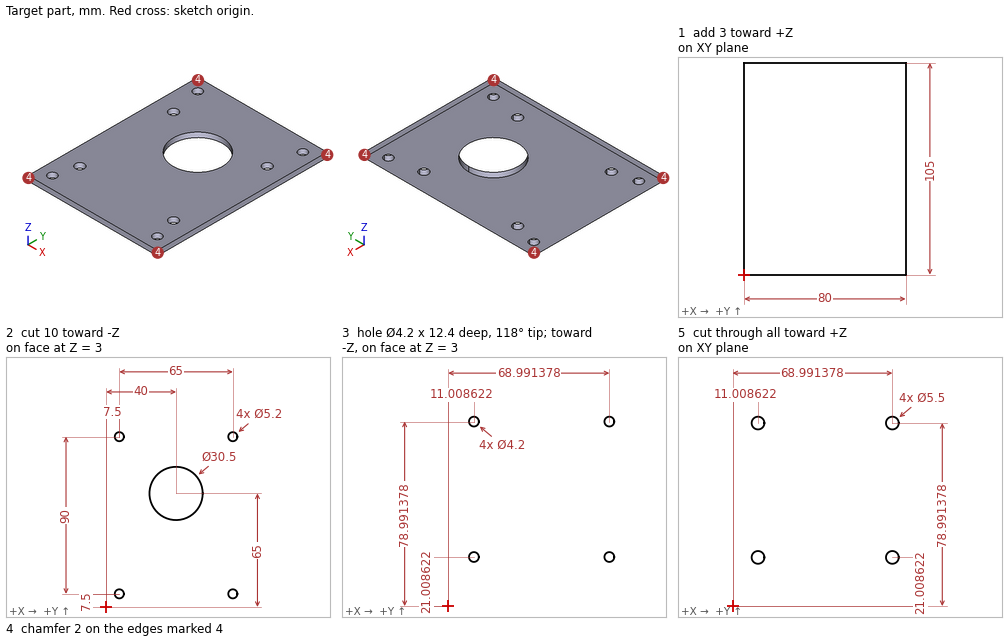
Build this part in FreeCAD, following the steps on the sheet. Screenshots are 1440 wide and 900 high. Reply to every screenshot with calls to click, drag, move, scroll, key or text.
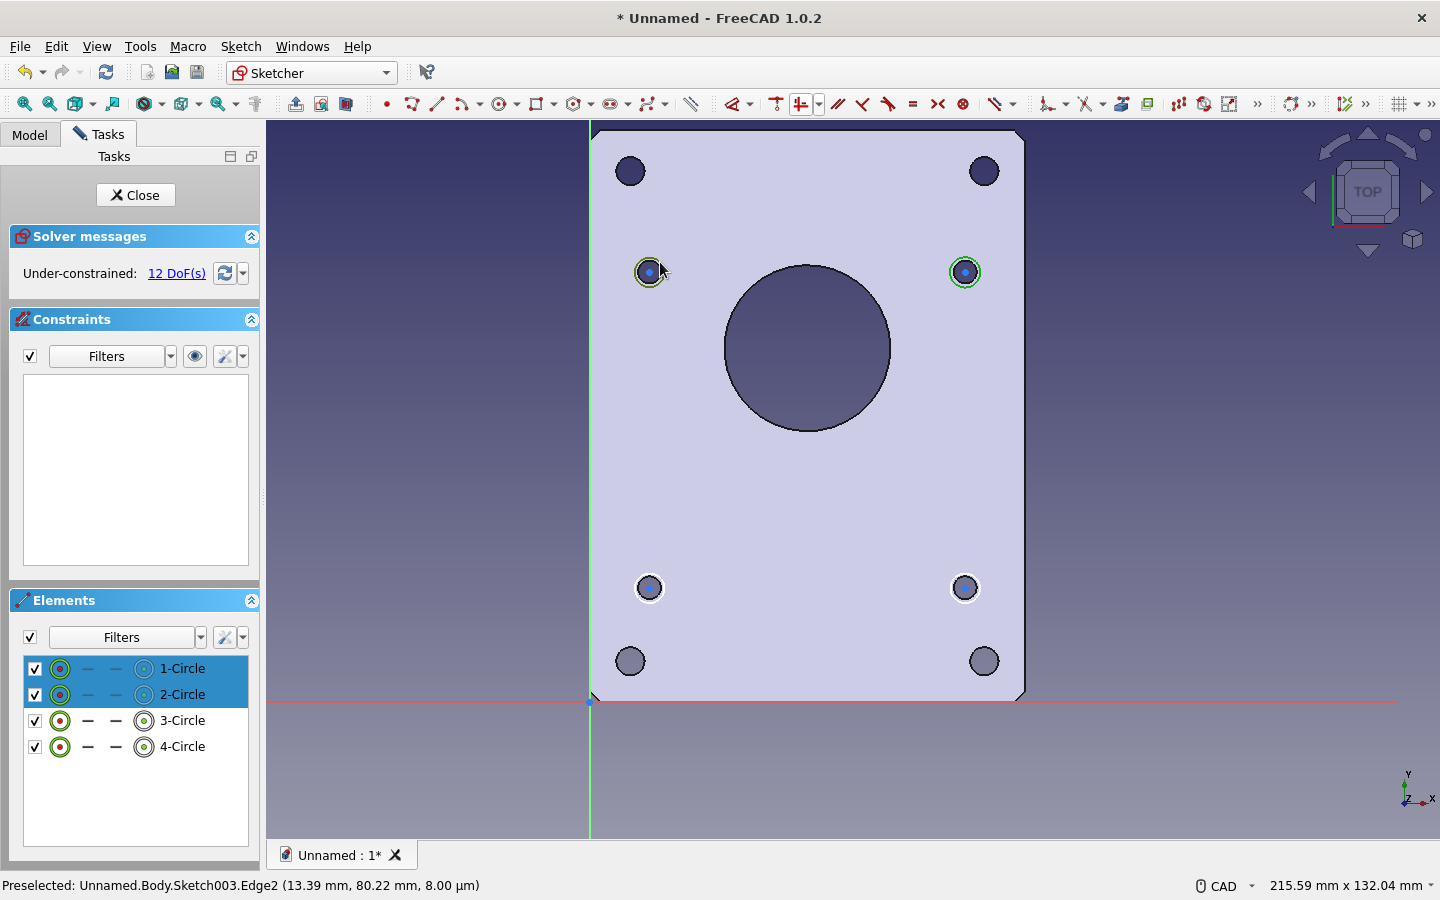
click(976, 578)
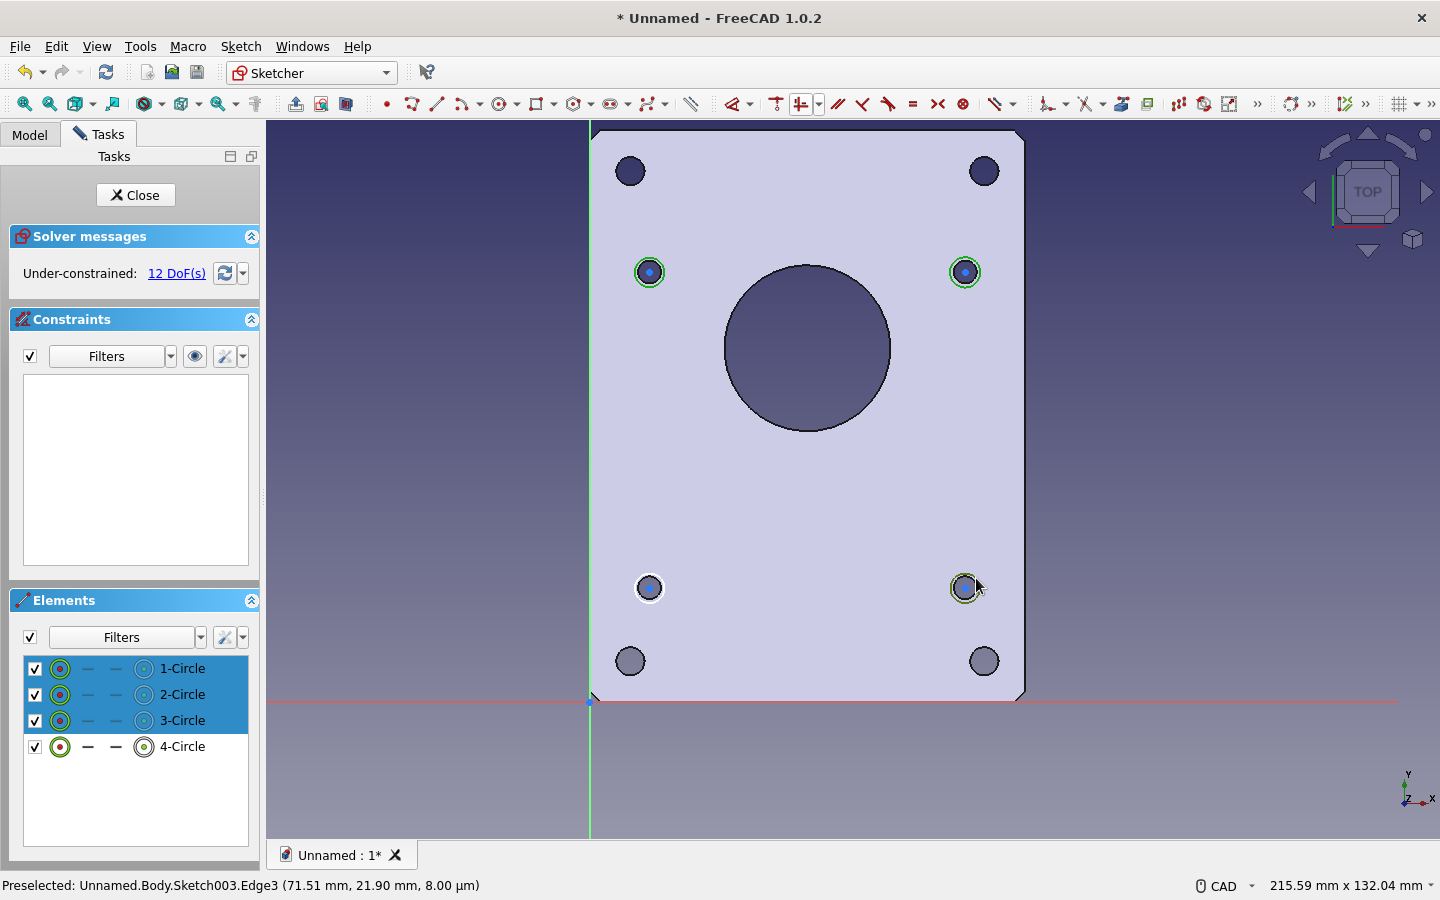
click(660, 578)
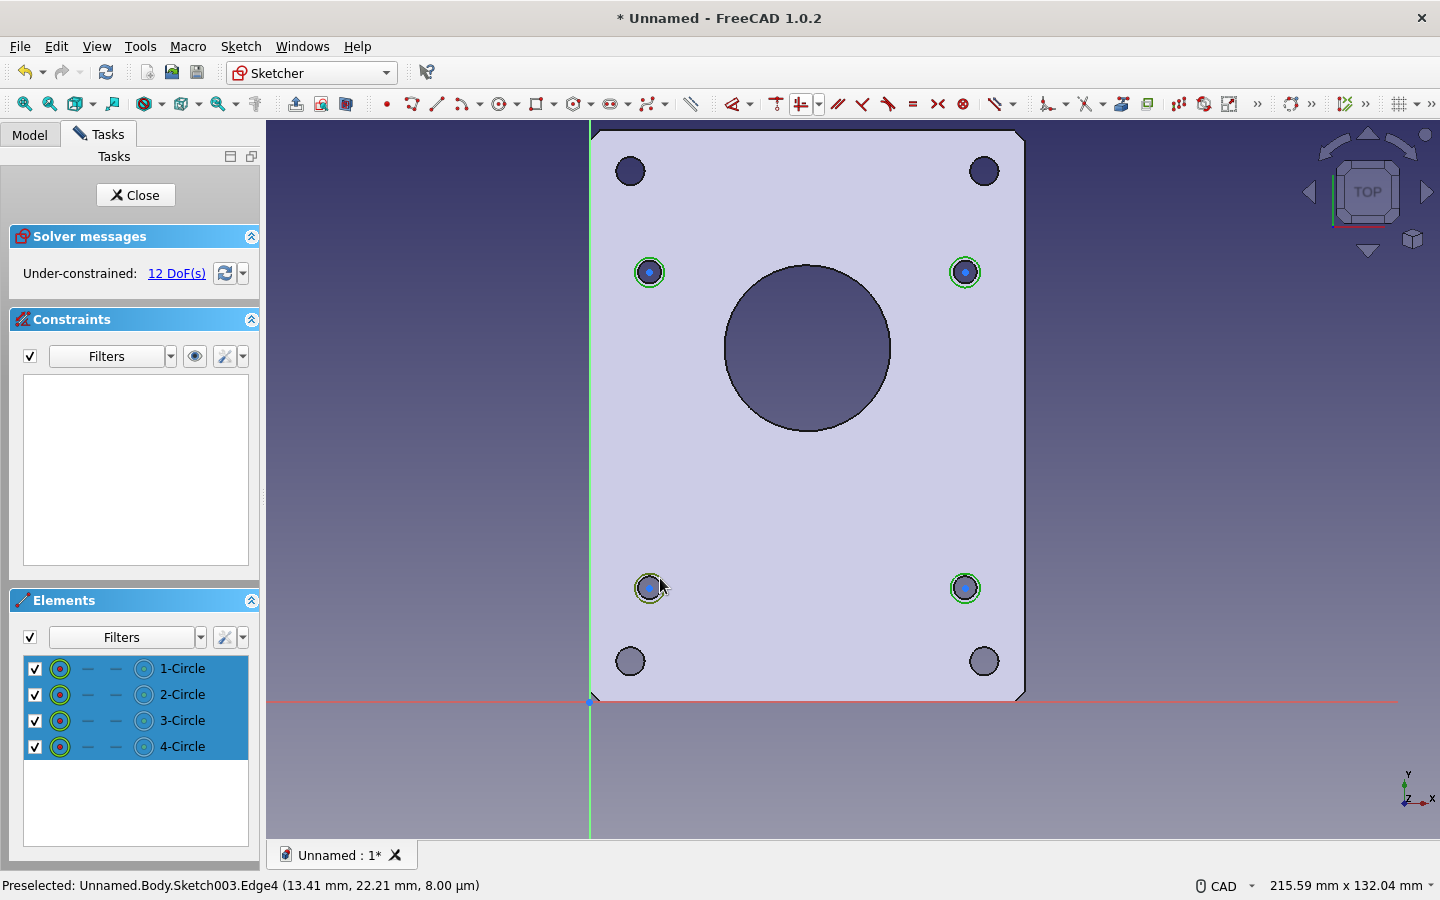
click(913, 104)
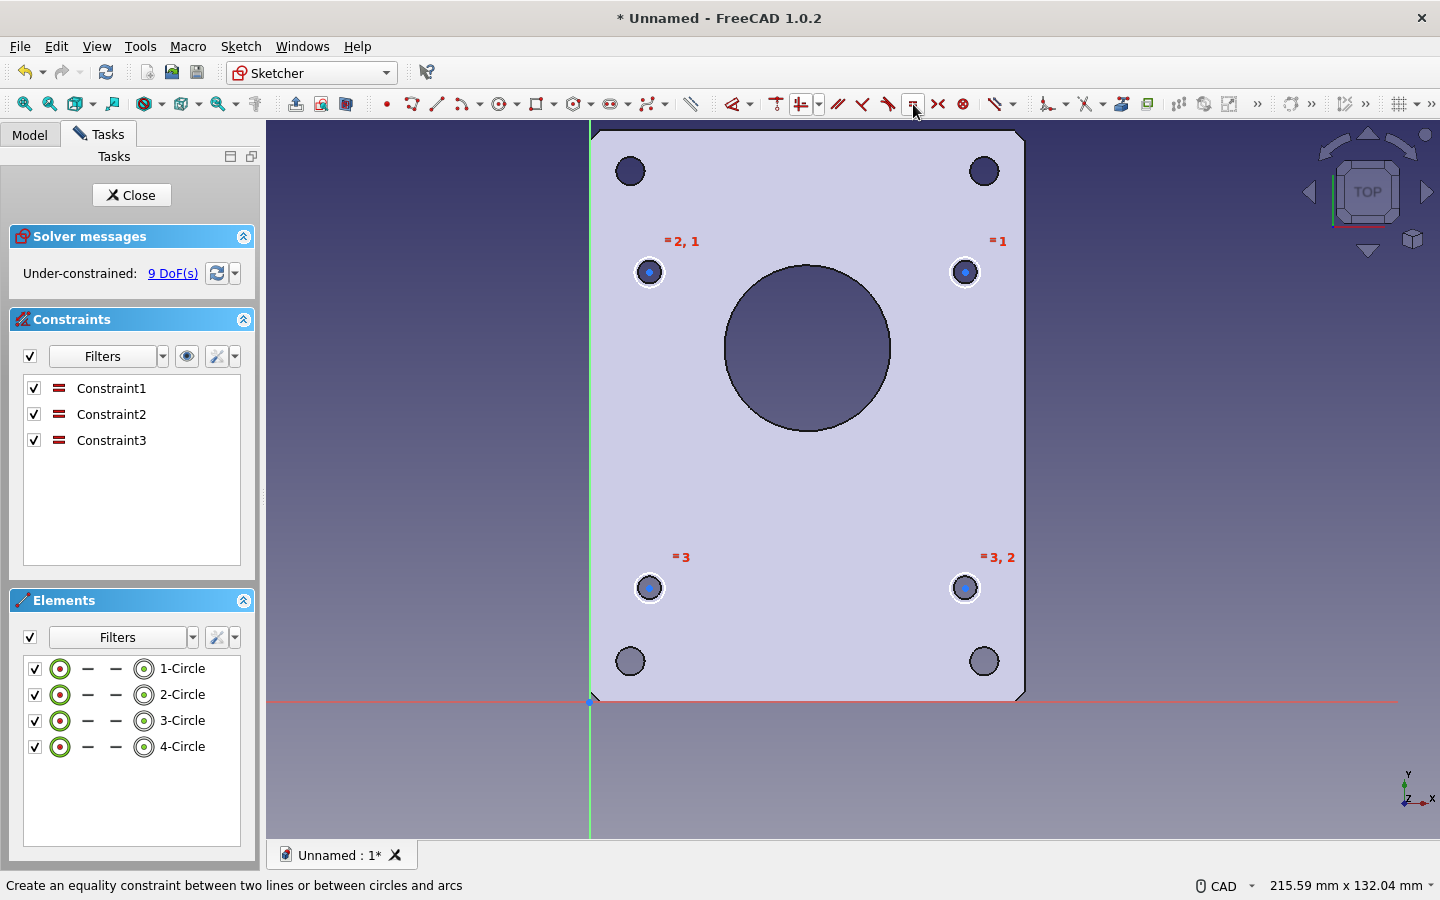
click(965, 272)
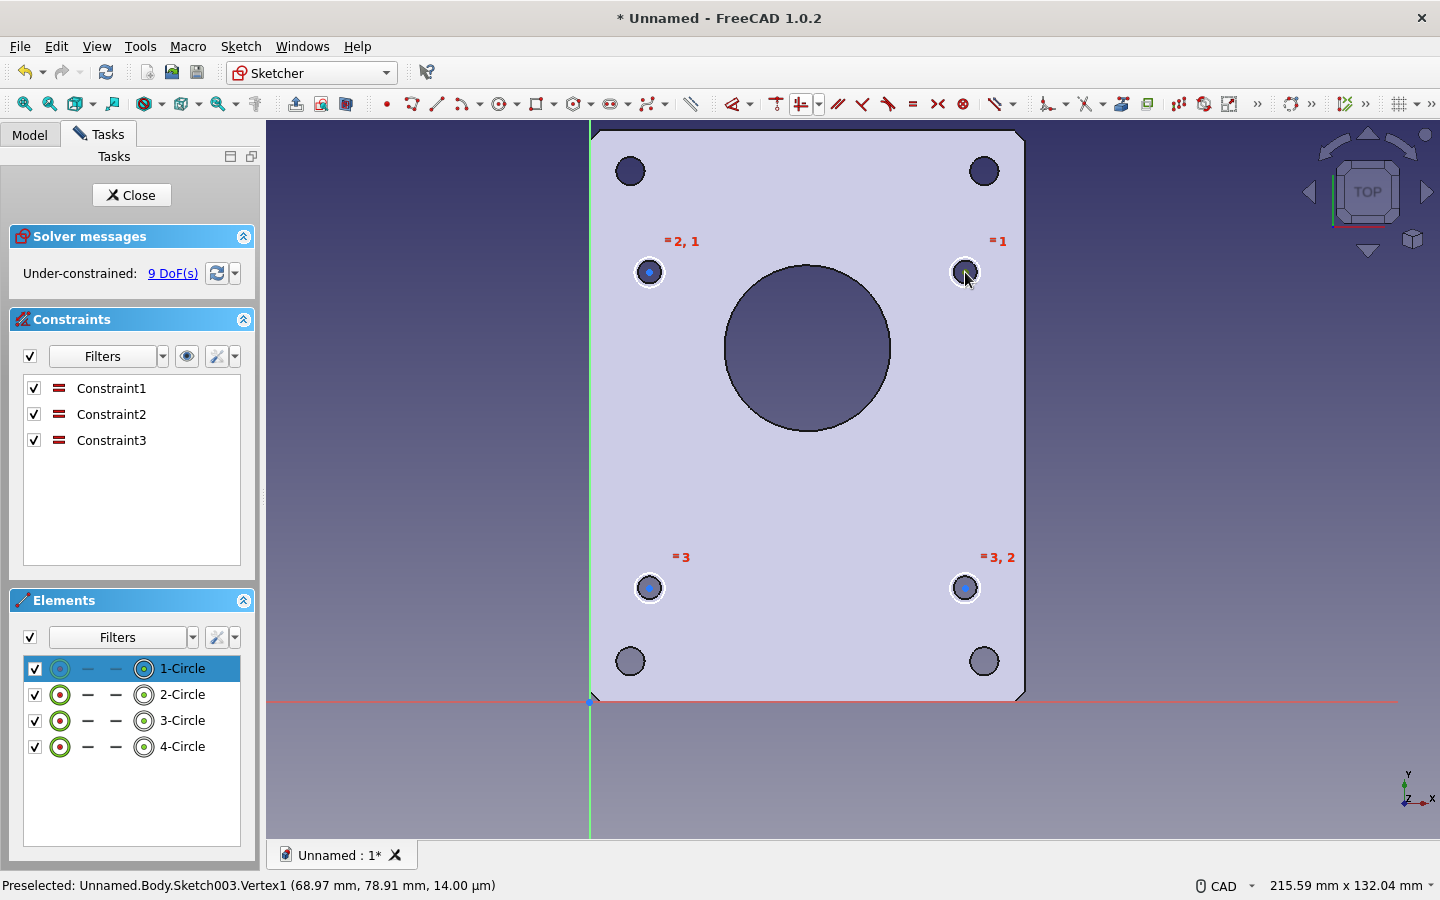
click(650, 272)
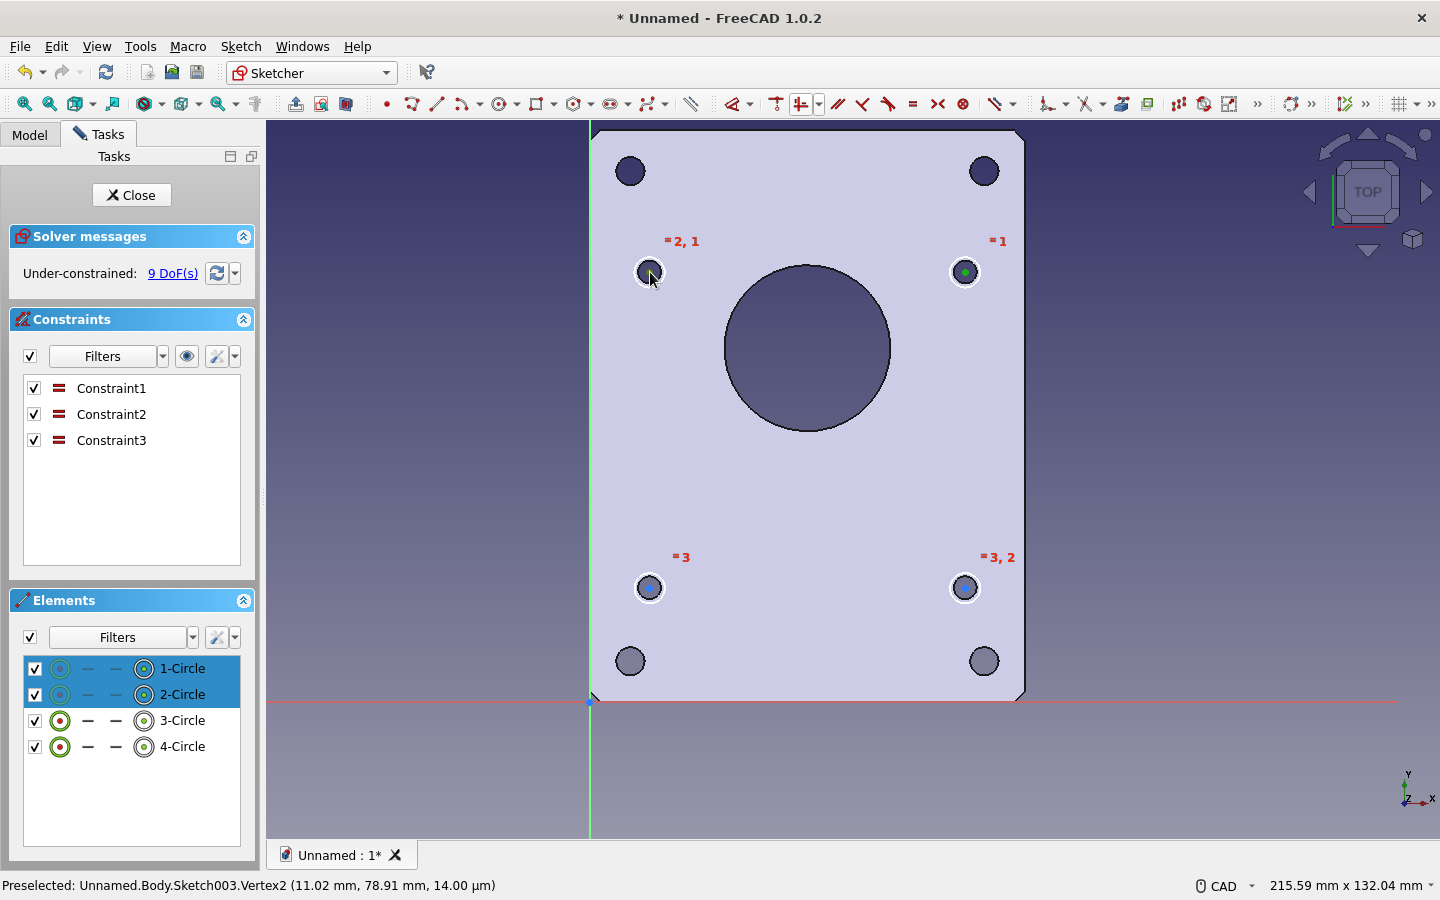
click(818, 104)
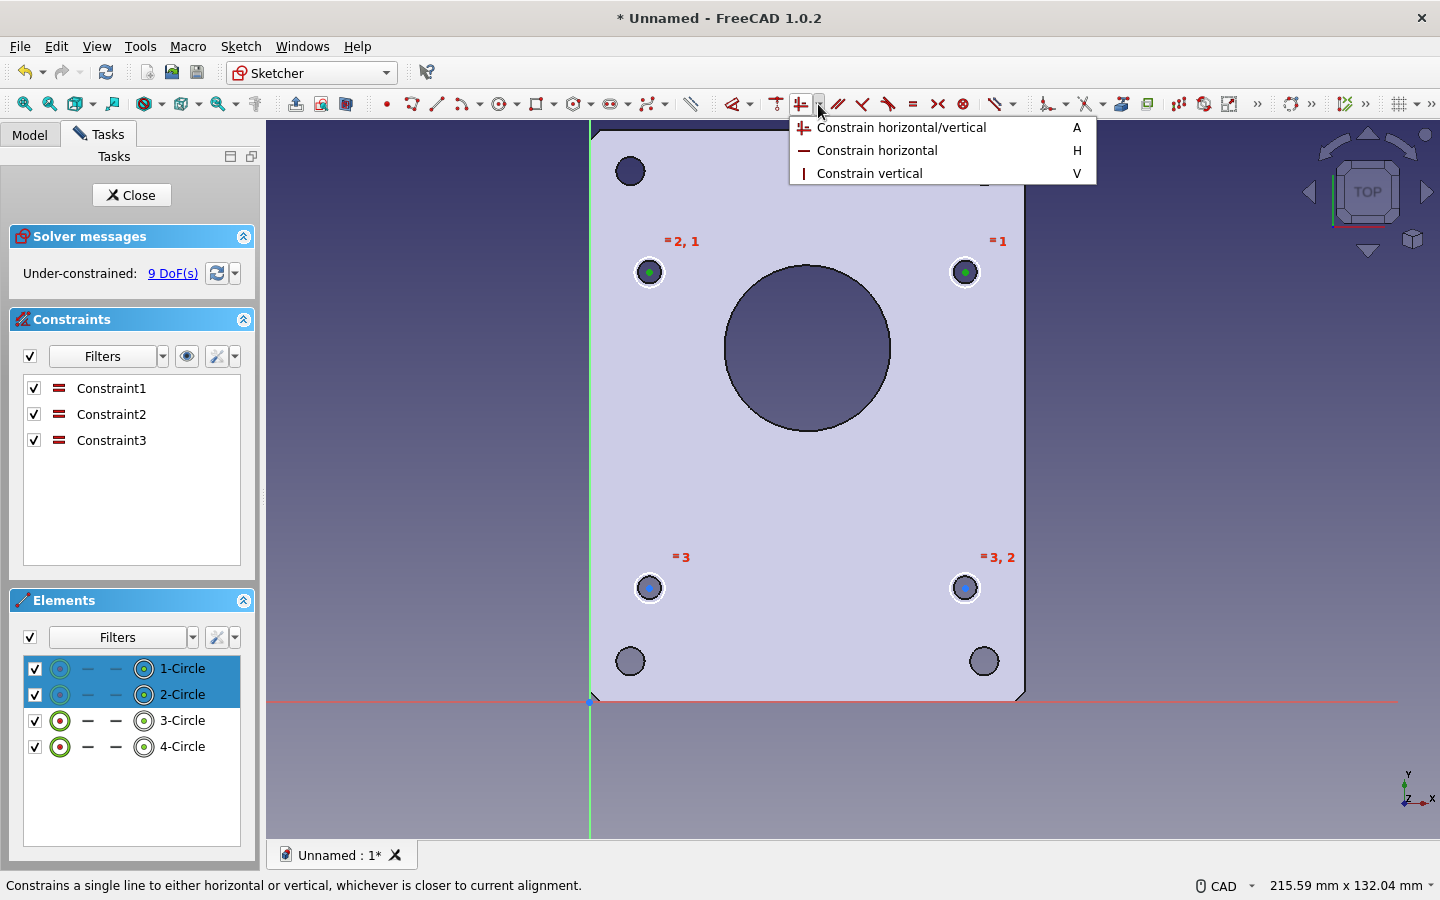
click(943, 150)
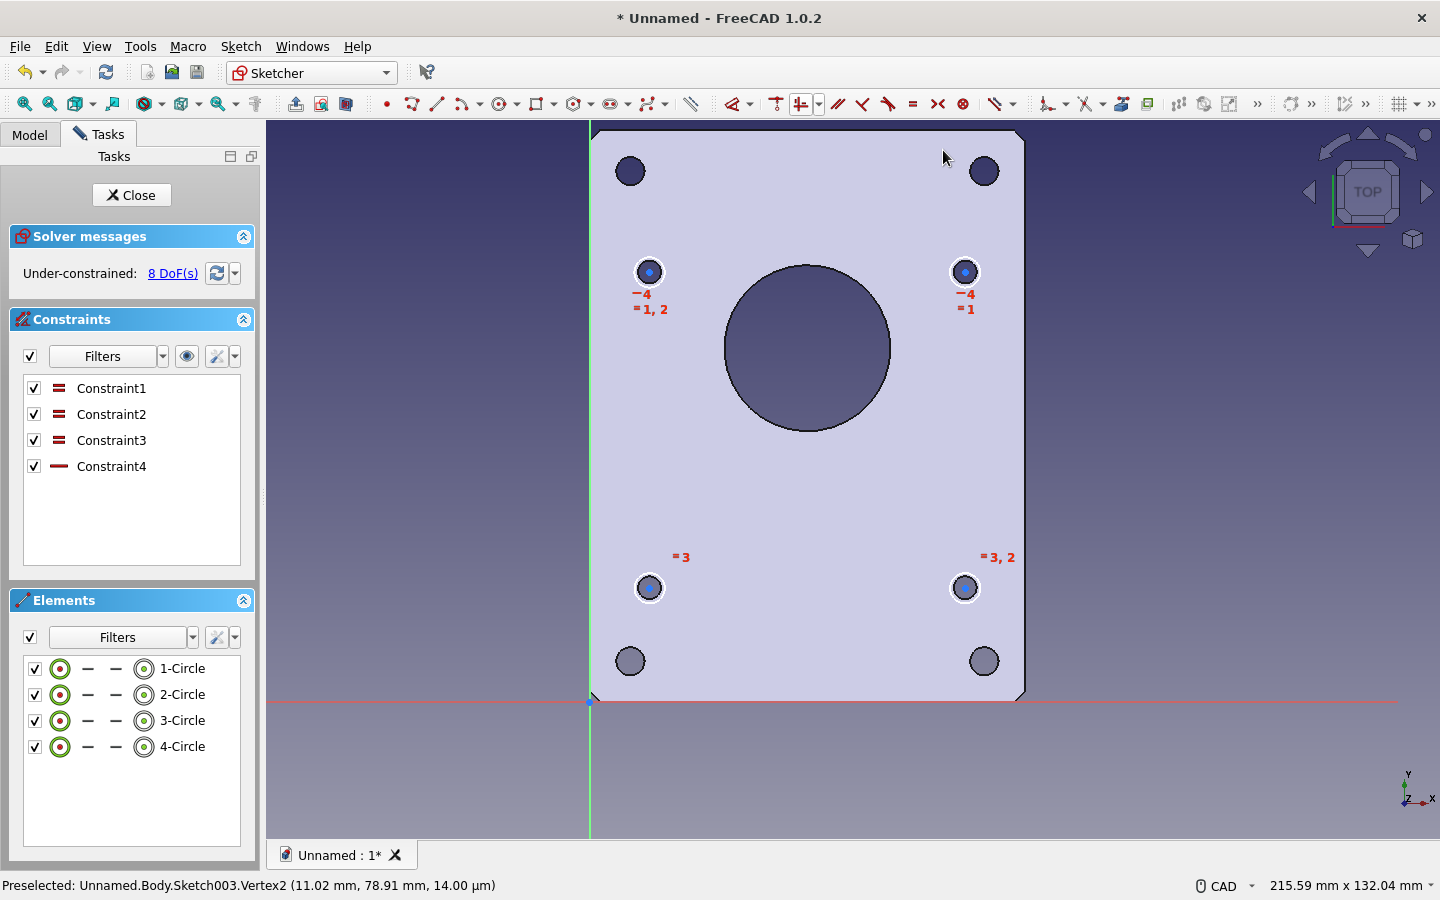
click(965, 272)